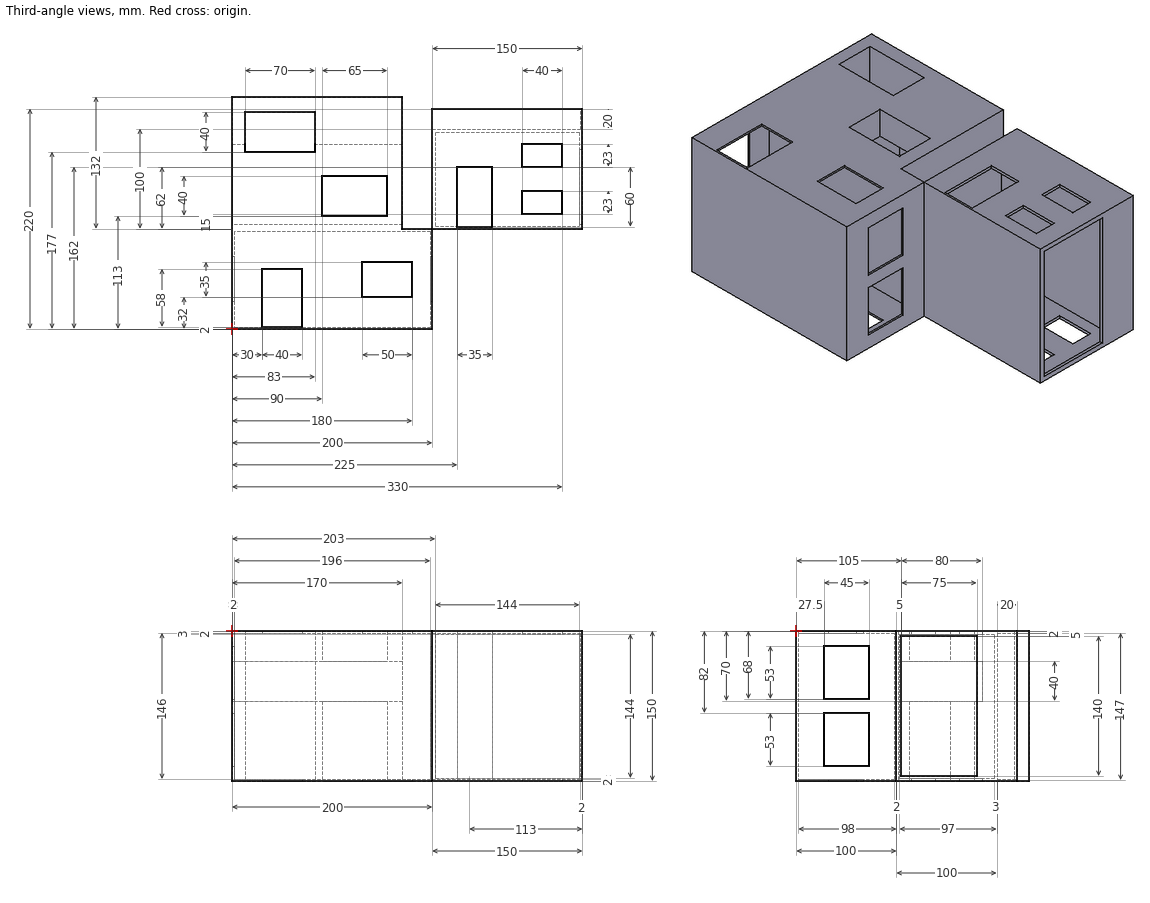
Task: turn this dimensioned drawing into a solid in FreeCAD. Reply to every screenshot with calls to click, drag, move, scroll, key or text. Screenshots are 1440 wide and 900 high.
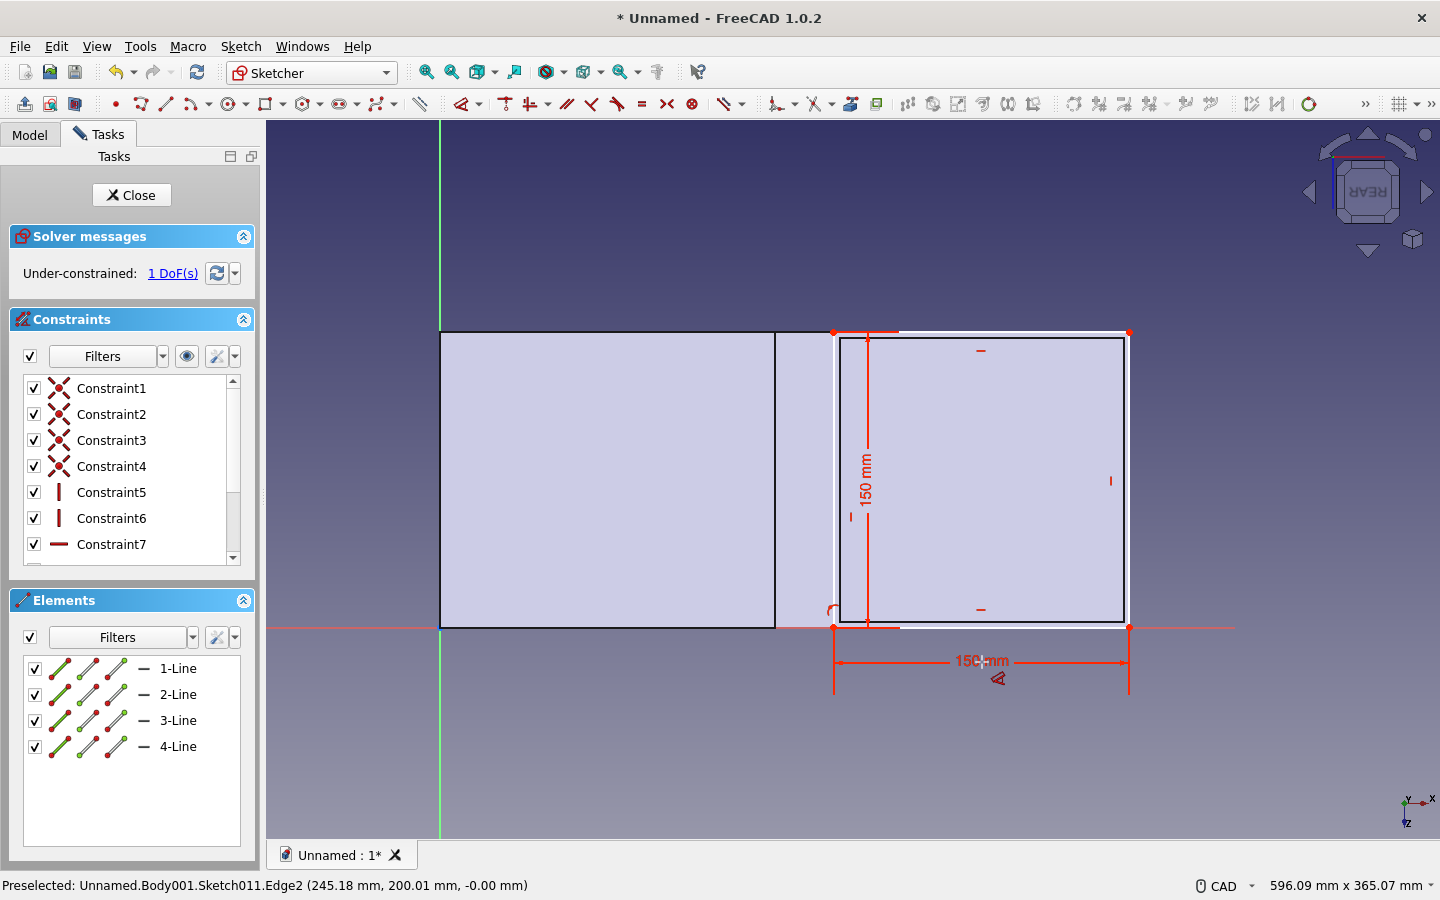
click(834, 332)
click(637, 662)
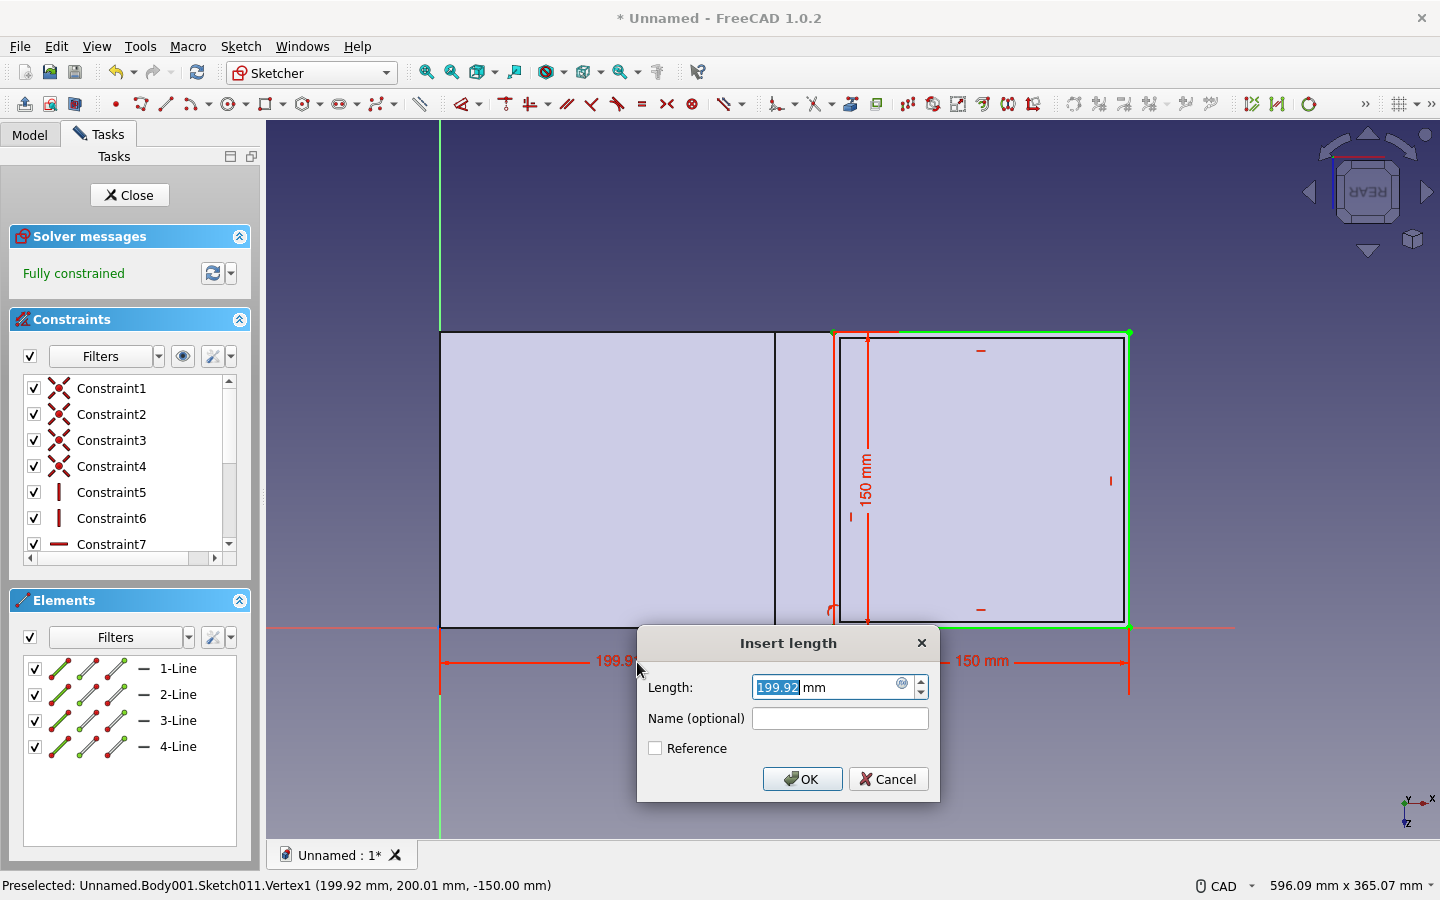
text(200)
key(Return)
key(Escape)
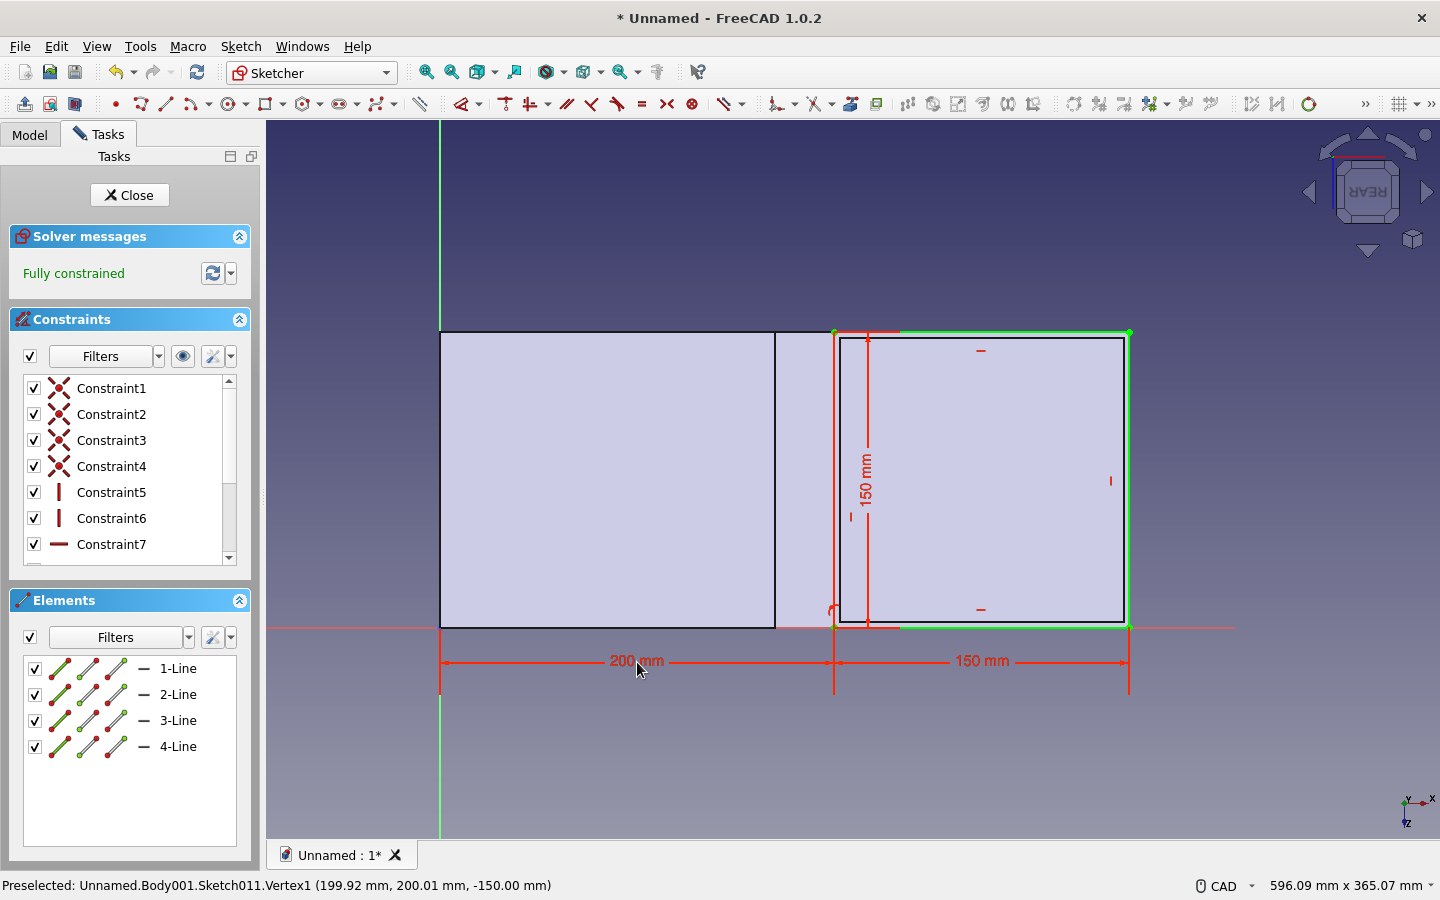
click(130, 195)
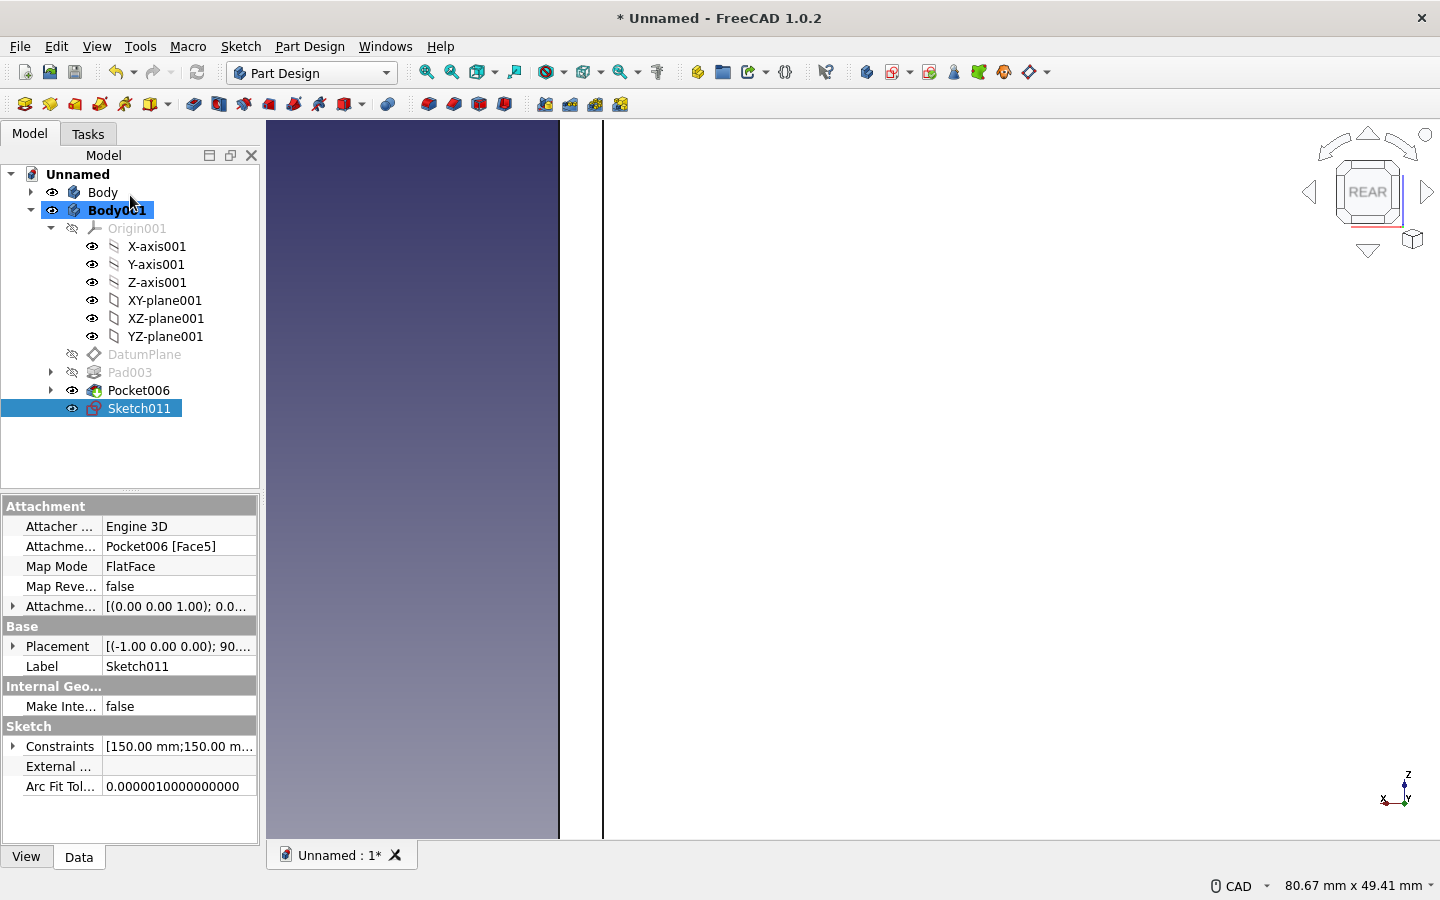
click(25, 104)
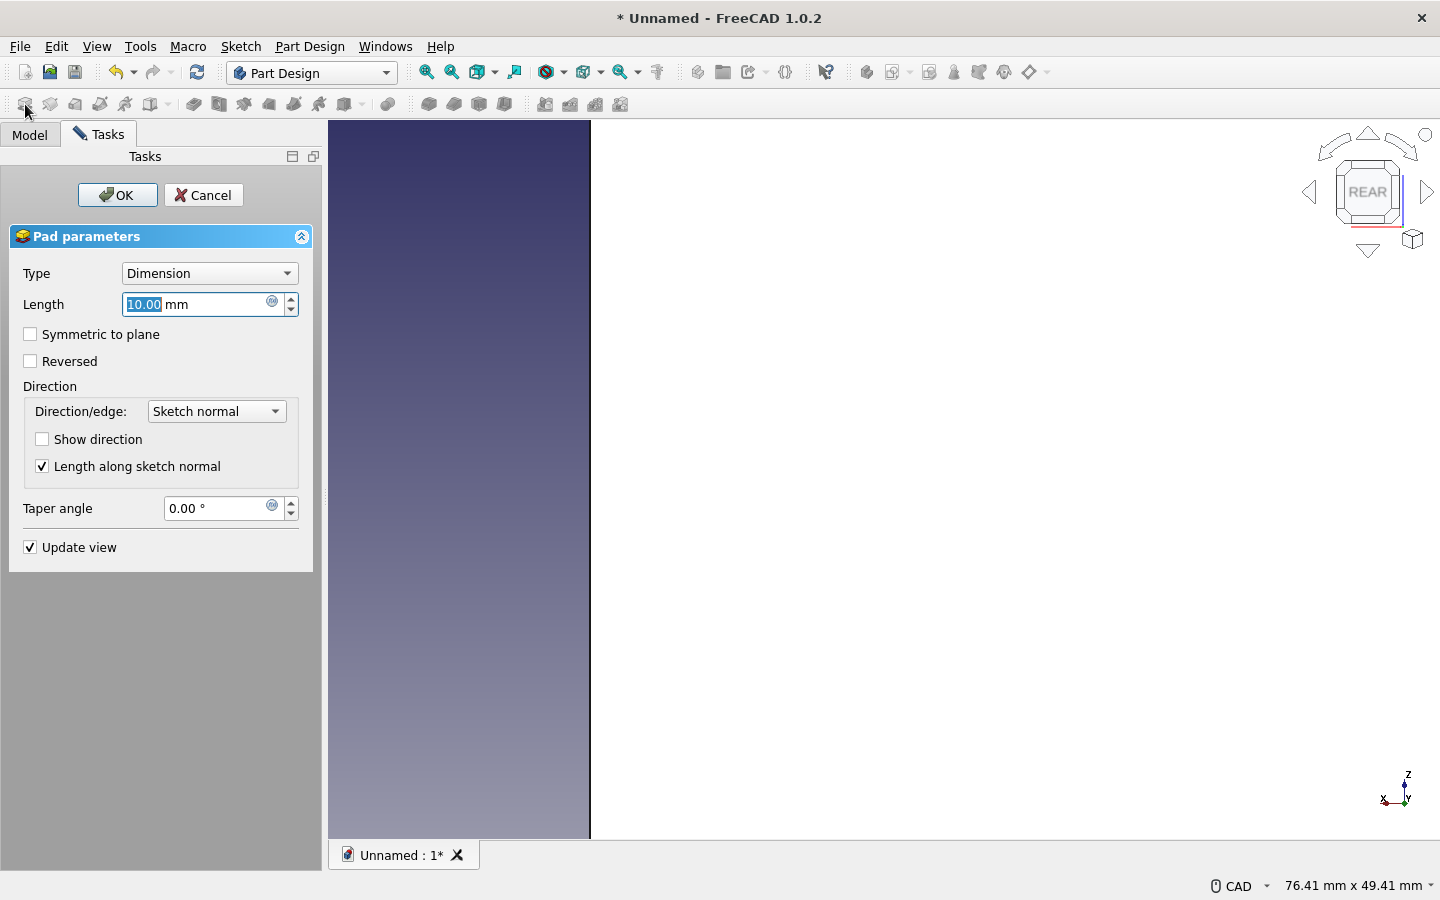
text(3)
key(Tab)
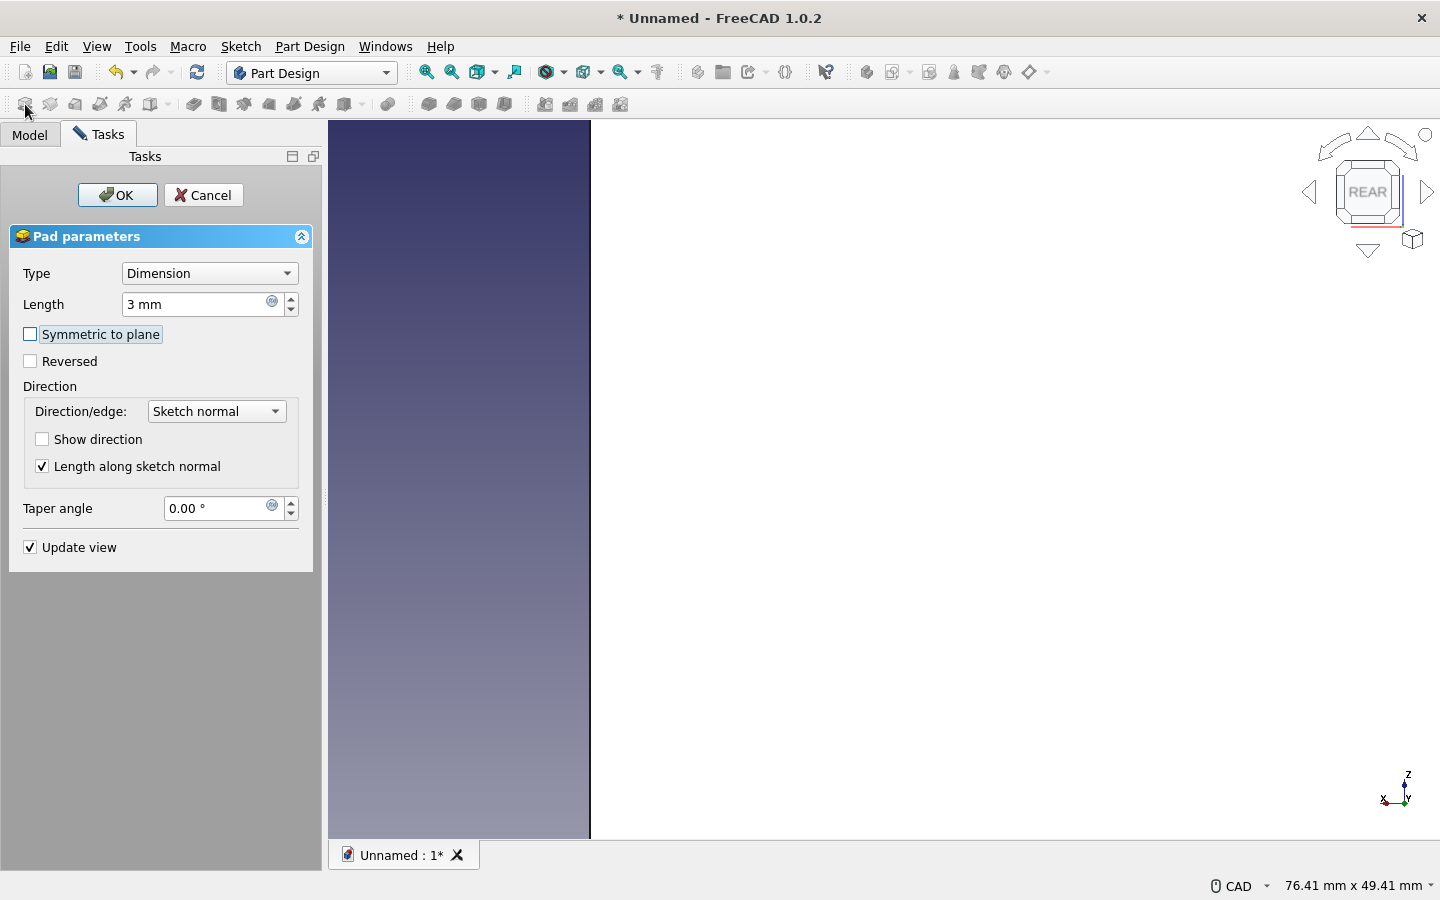
click(31, 361)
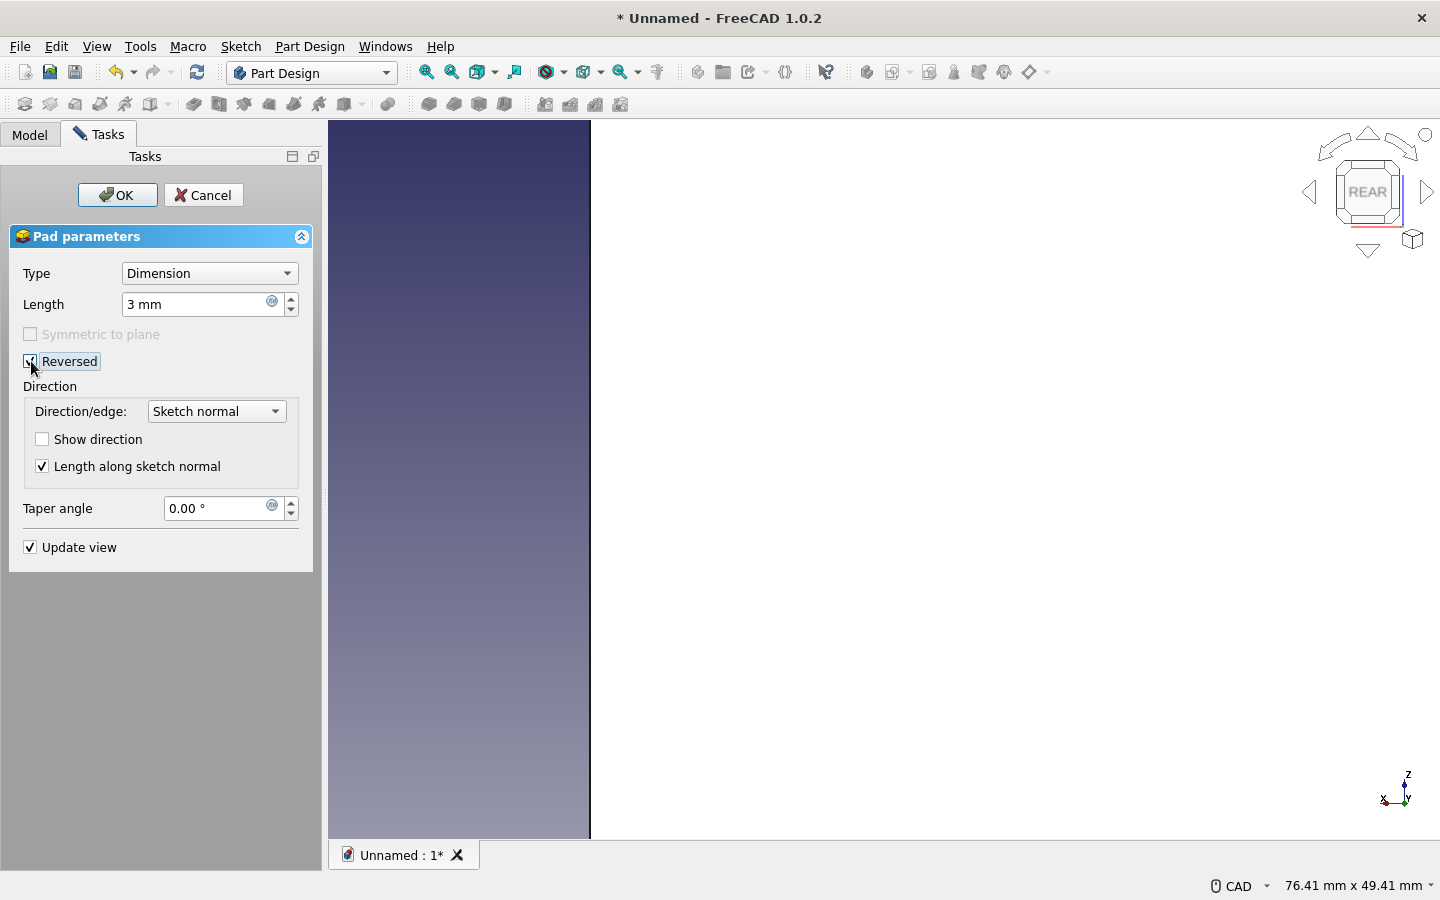
click(118, 195)